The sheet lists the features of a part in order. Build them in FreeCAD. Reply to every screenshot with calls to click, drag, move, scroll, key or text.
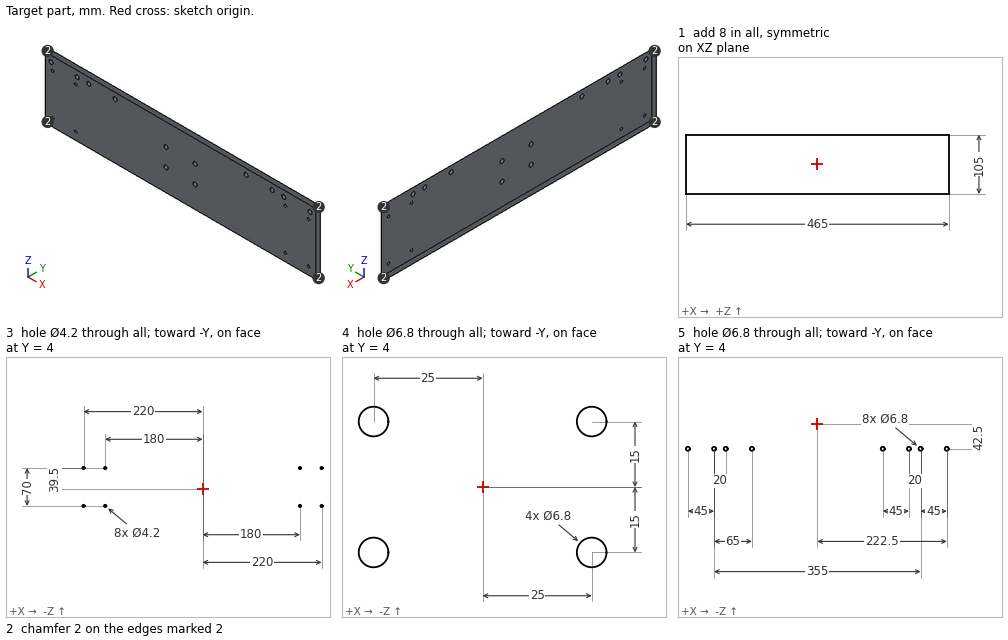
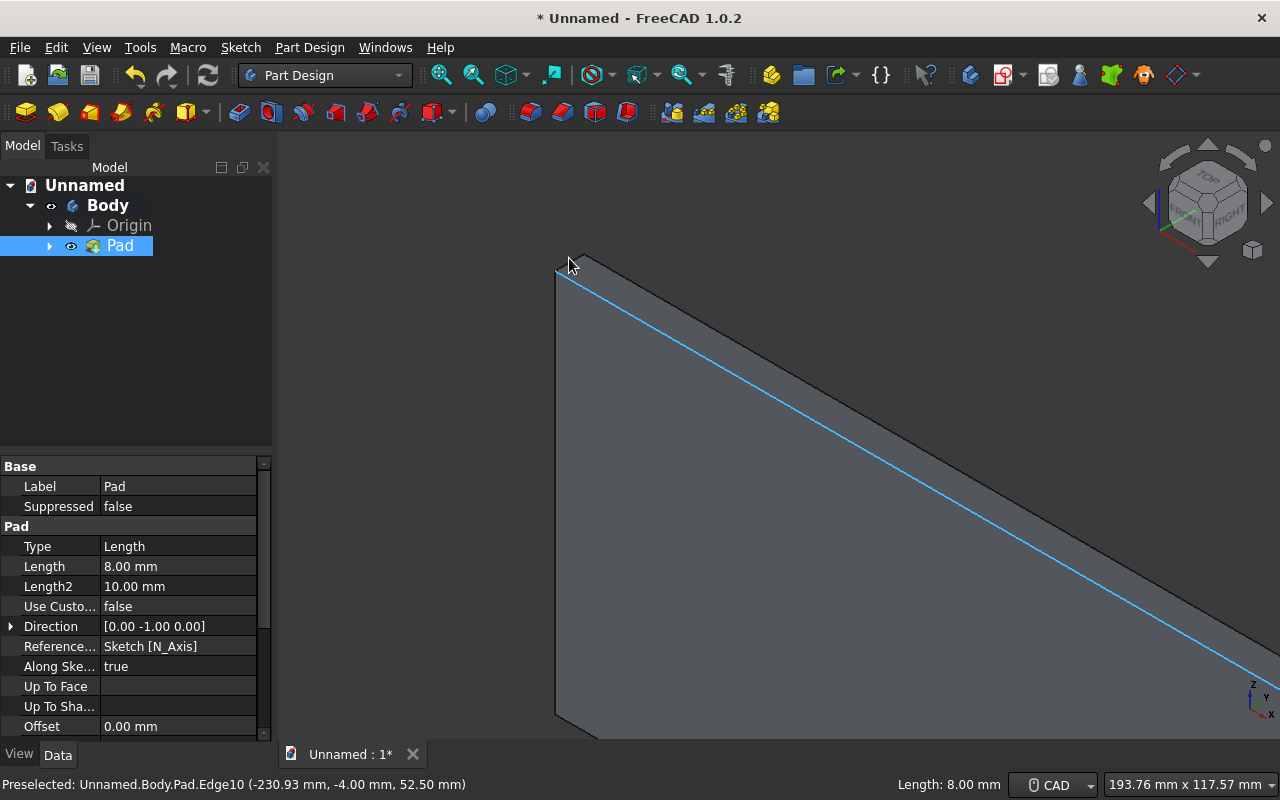
click(442, 76)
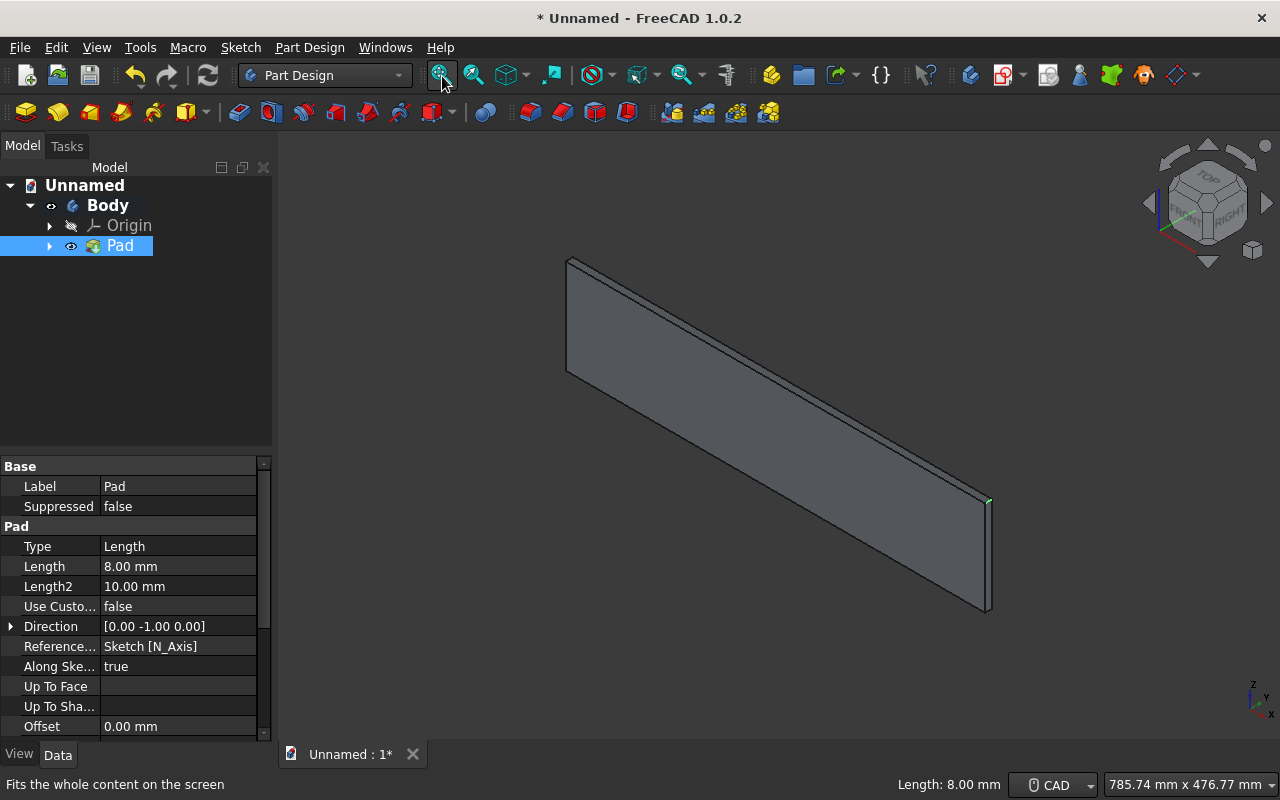
key(2)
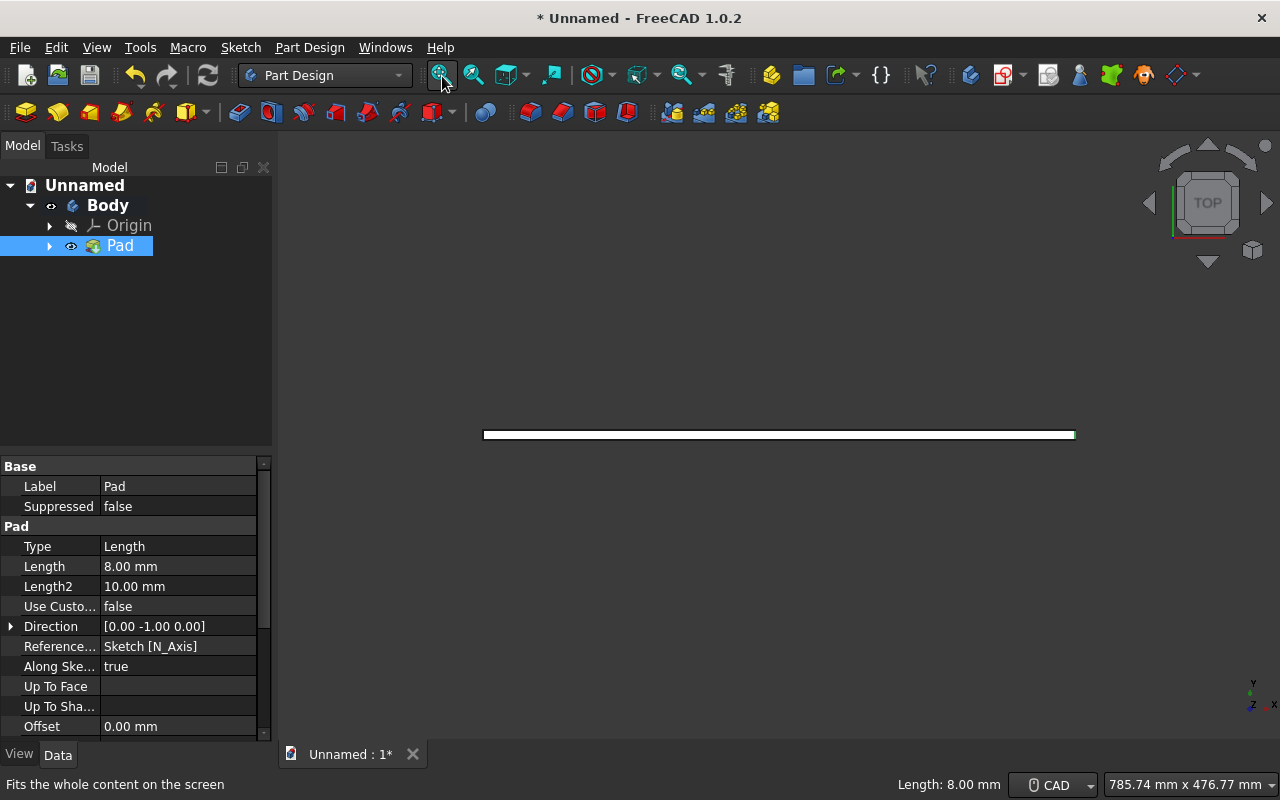
click(483, 435, ctrl)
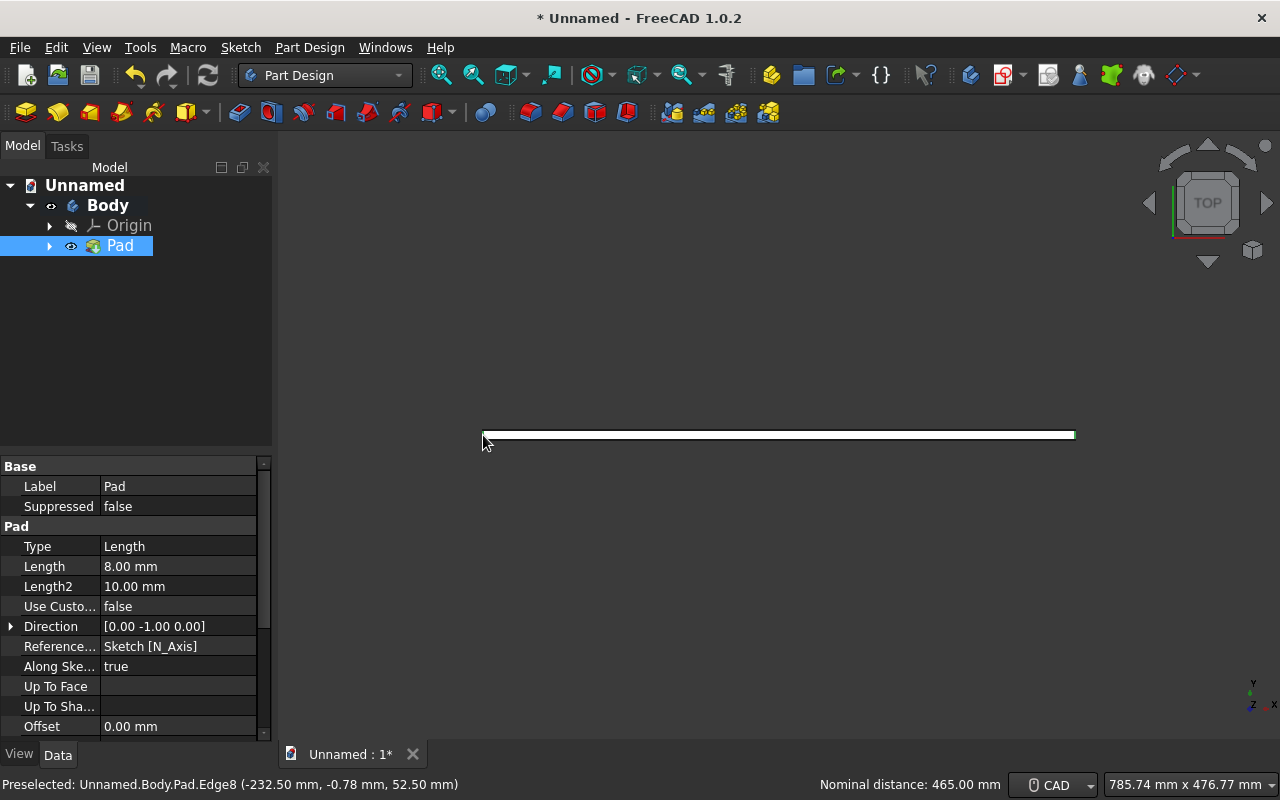
scroll(483, 434, up, 7)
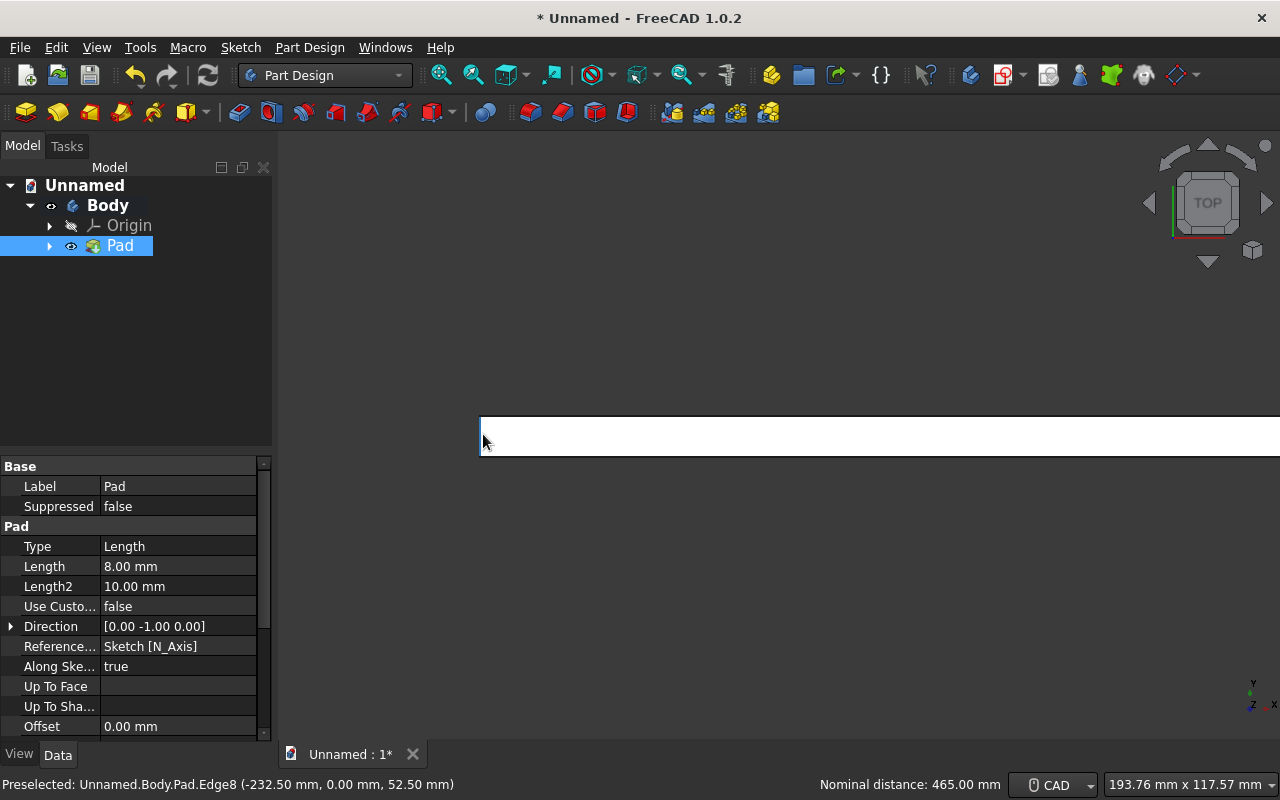
click(442, 76)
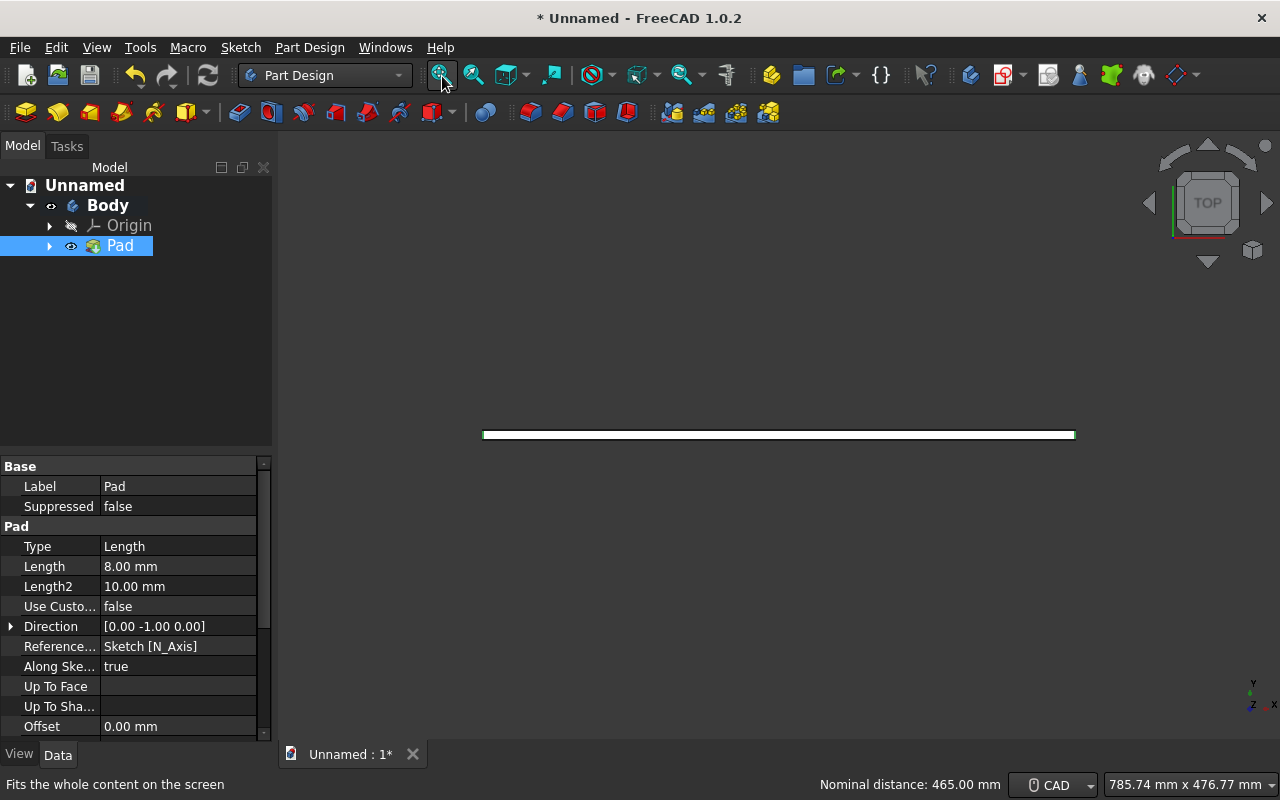
key(1)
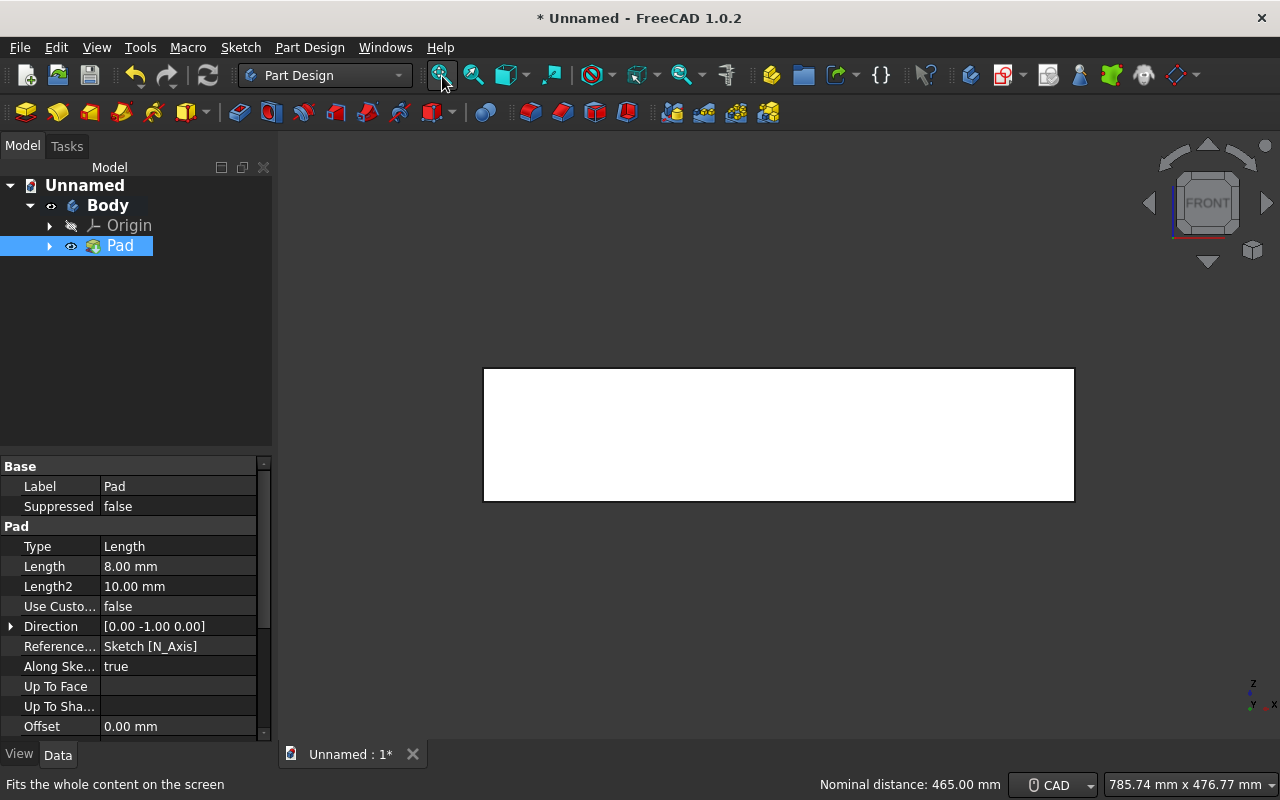
scroll(483, 501, up, 7)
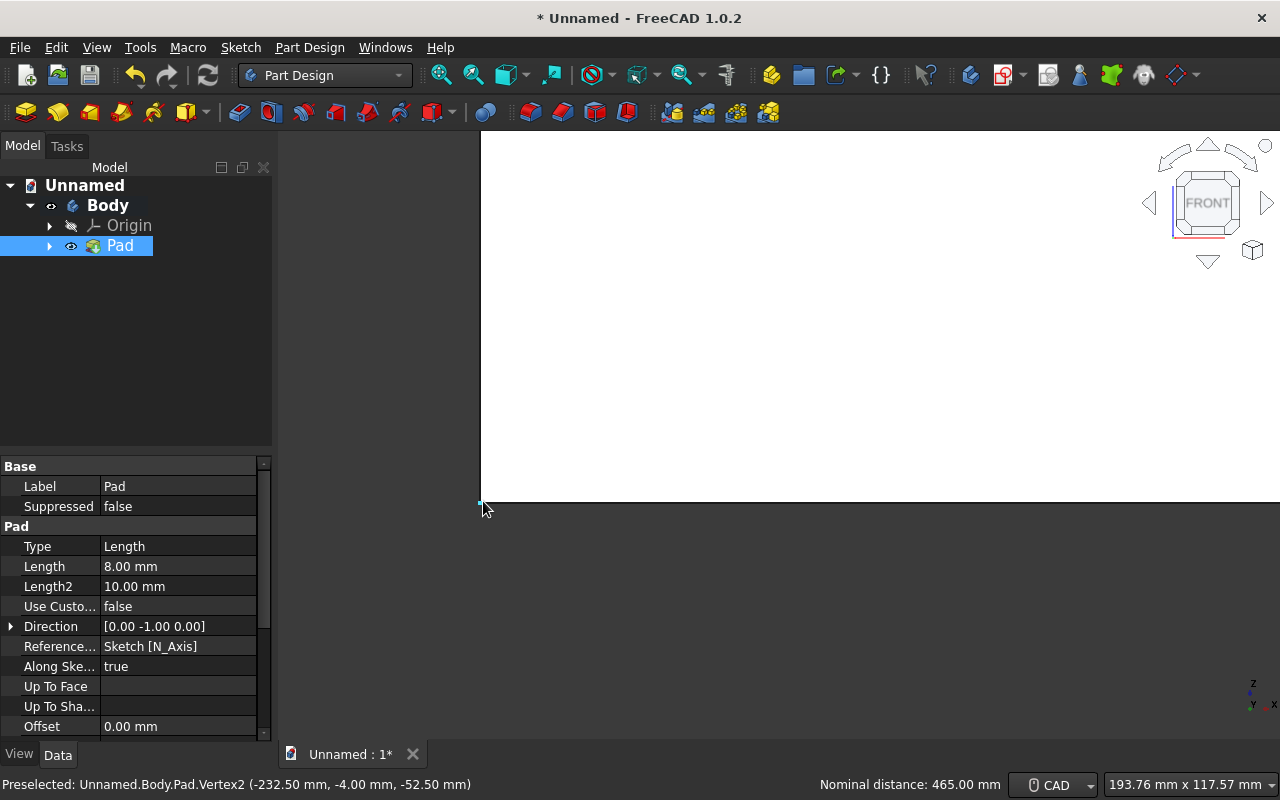
click(442, 76)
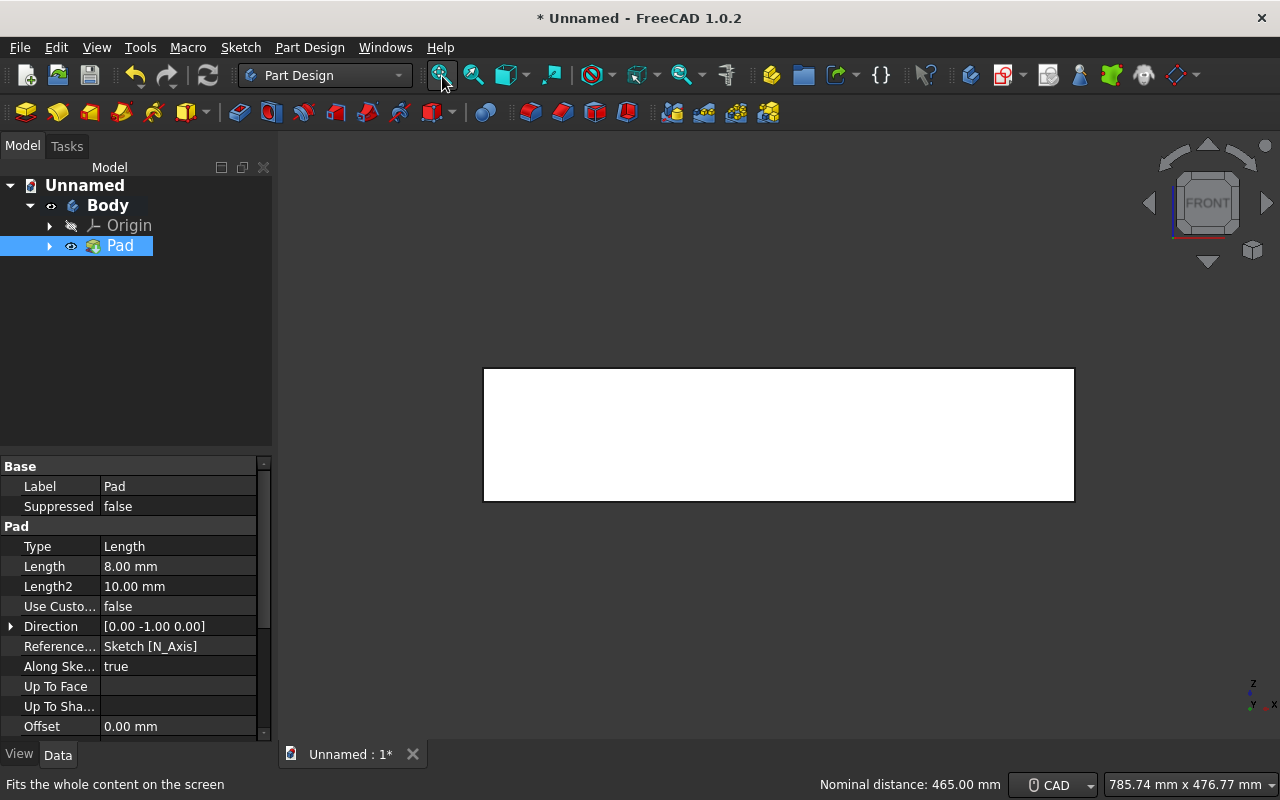
key(3)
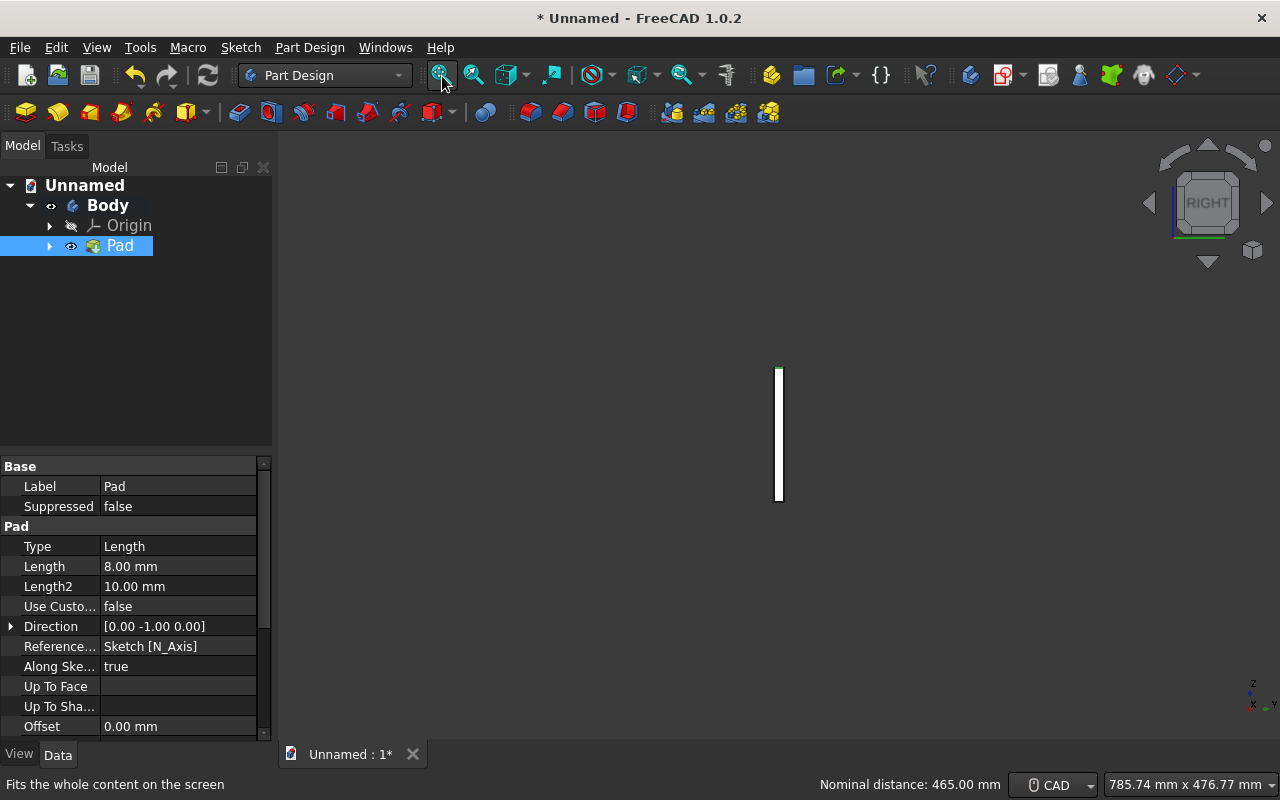
click(442, 76)